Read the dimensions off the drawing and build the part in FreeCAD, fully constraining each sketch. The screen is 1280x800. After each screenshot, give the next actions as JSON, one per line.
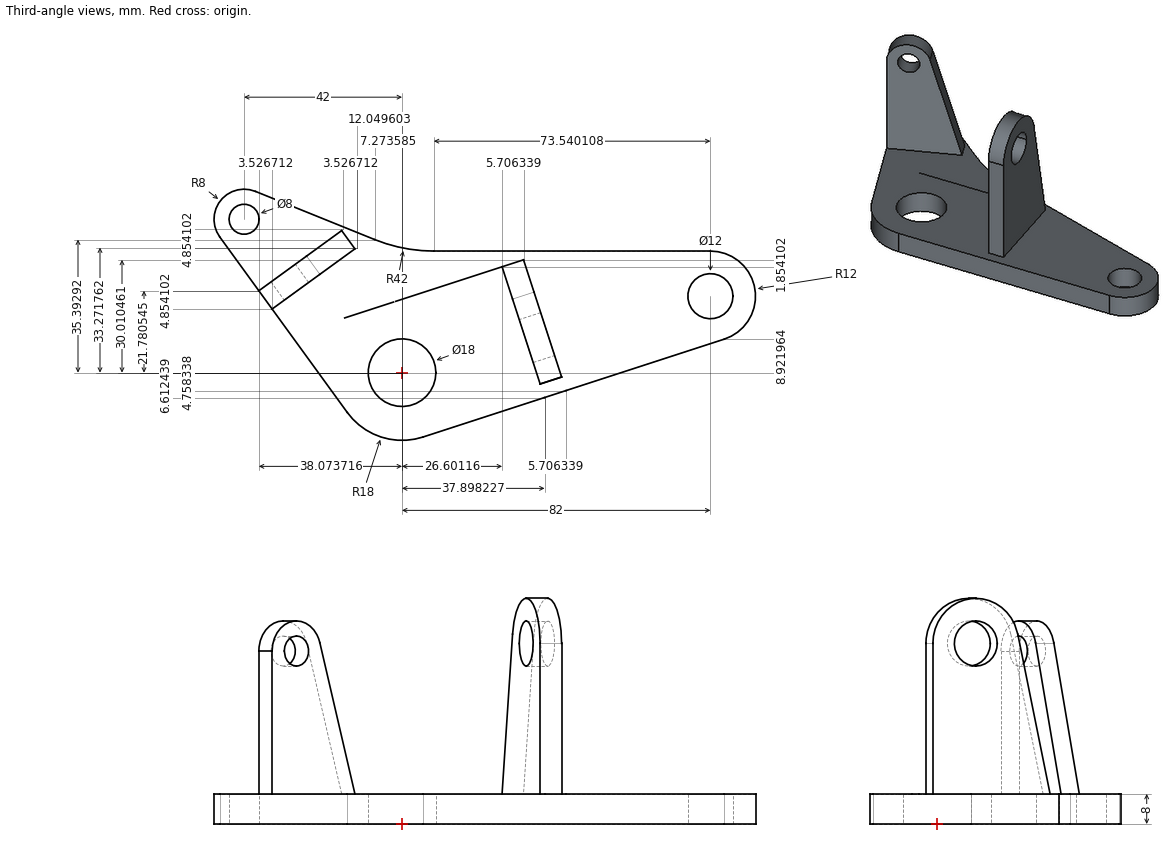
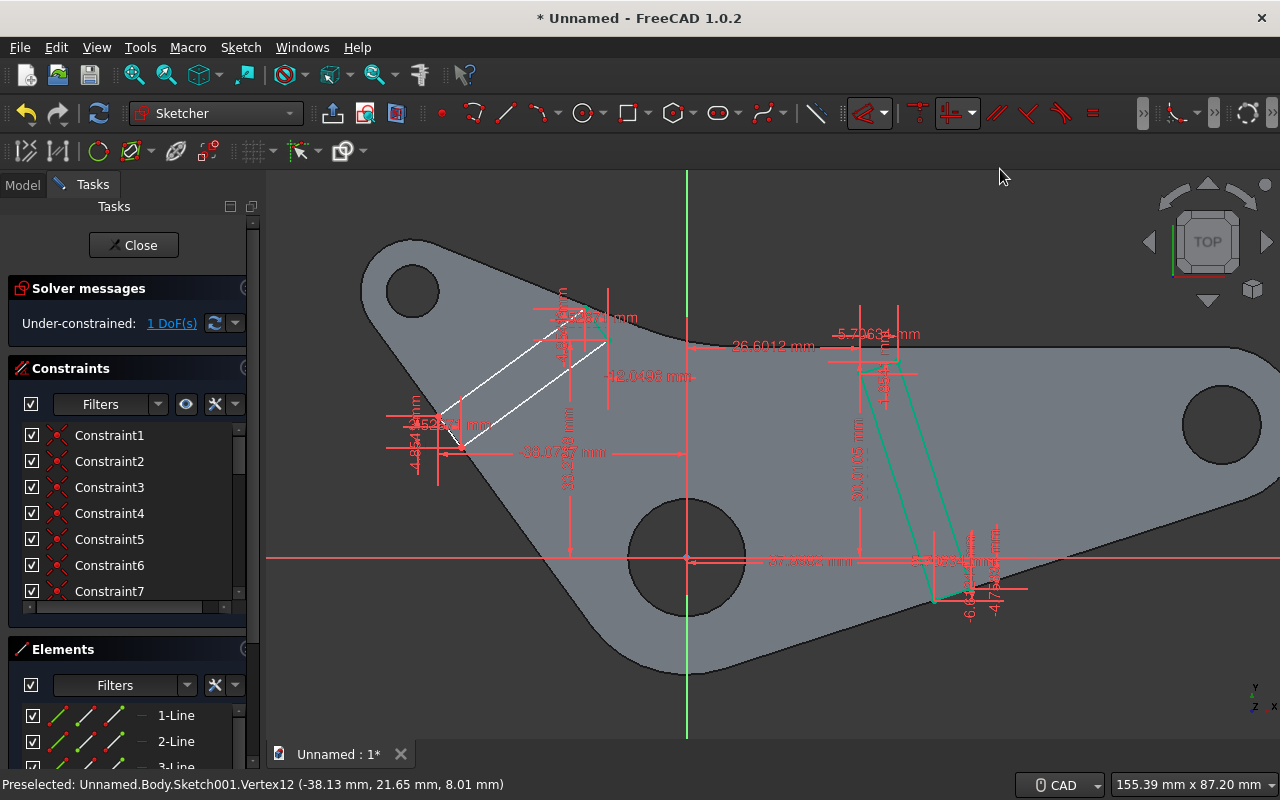
{"action": "left_click", "coordinate": [438, 416]}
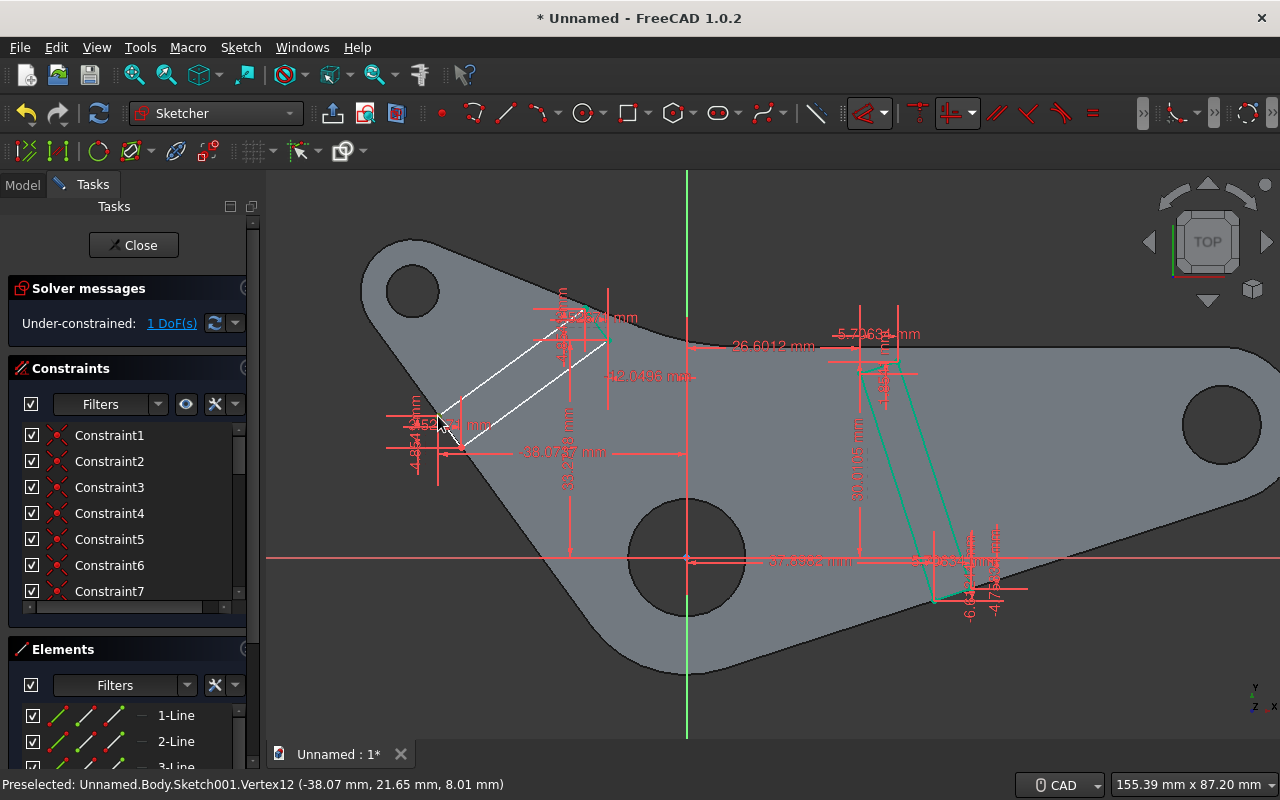
{"action": "key", "text": "i"}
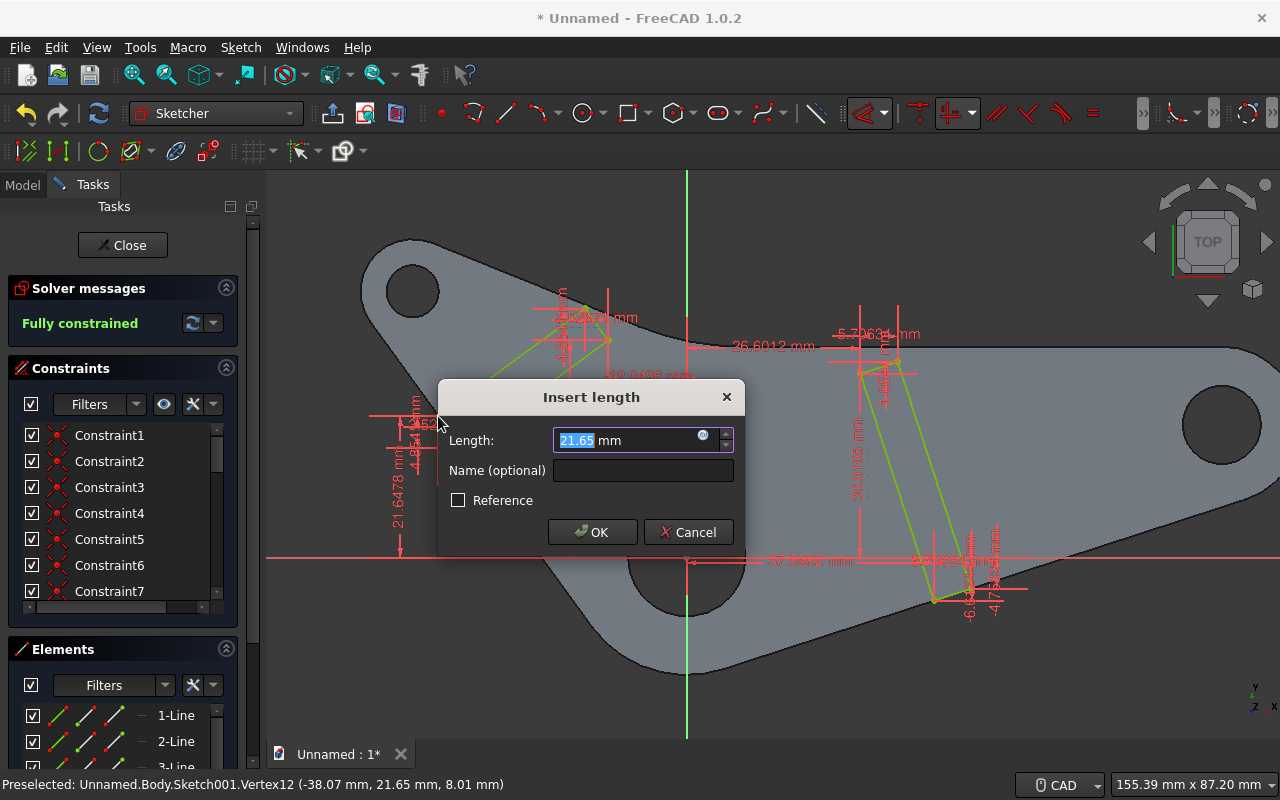
{"action": "type", "text": "21.780545"}
{"action": "key", "text": "Return"}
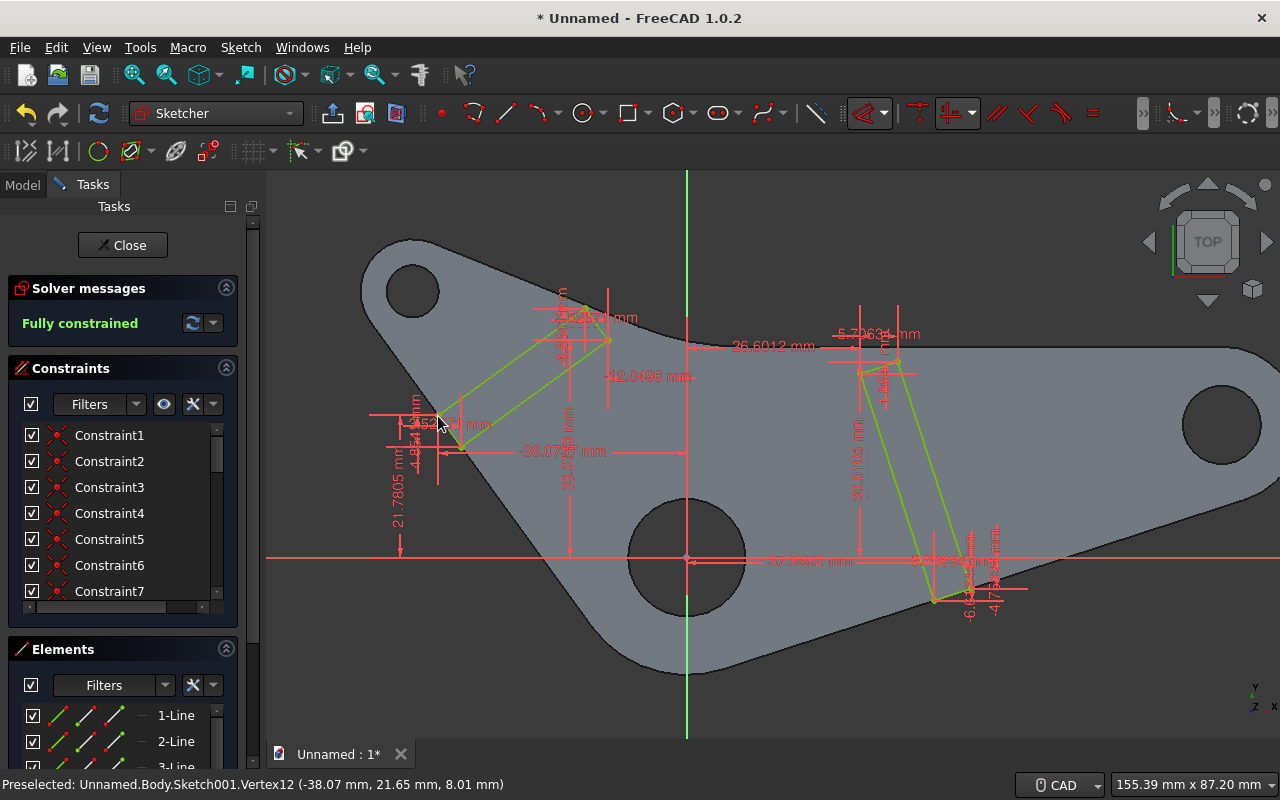
{"action": "left_click", "coordinate": [123, 245]}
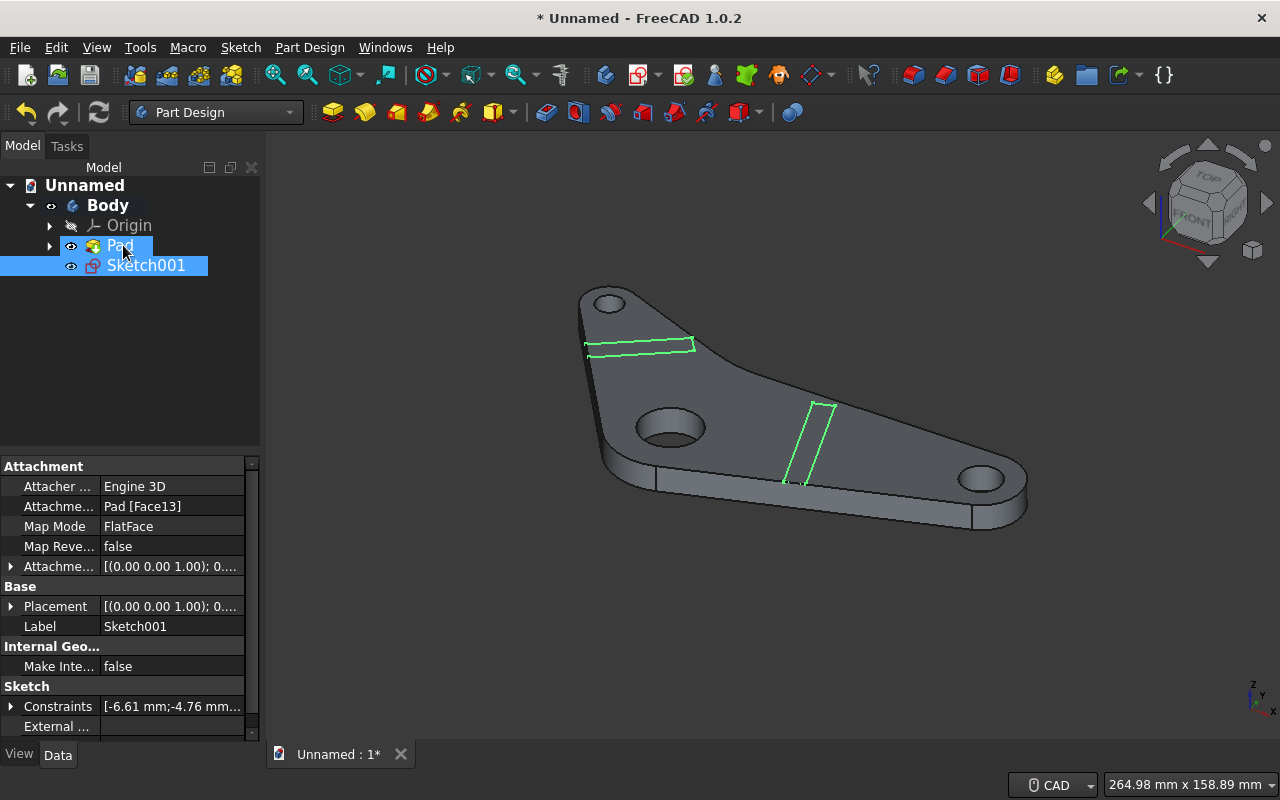
{"action": "left_click", "coordinate": [334, 112]}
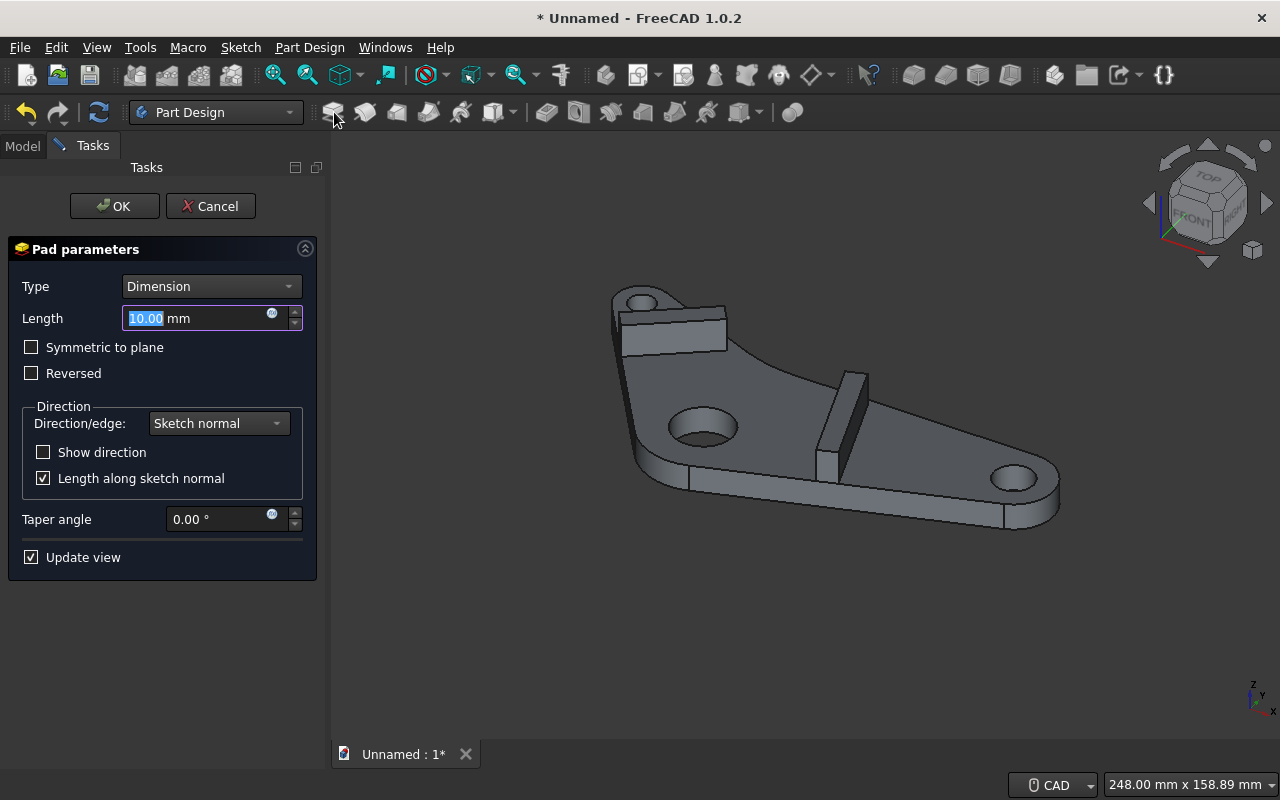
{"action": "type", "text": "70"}
{"action": "key", "text": "Tab"}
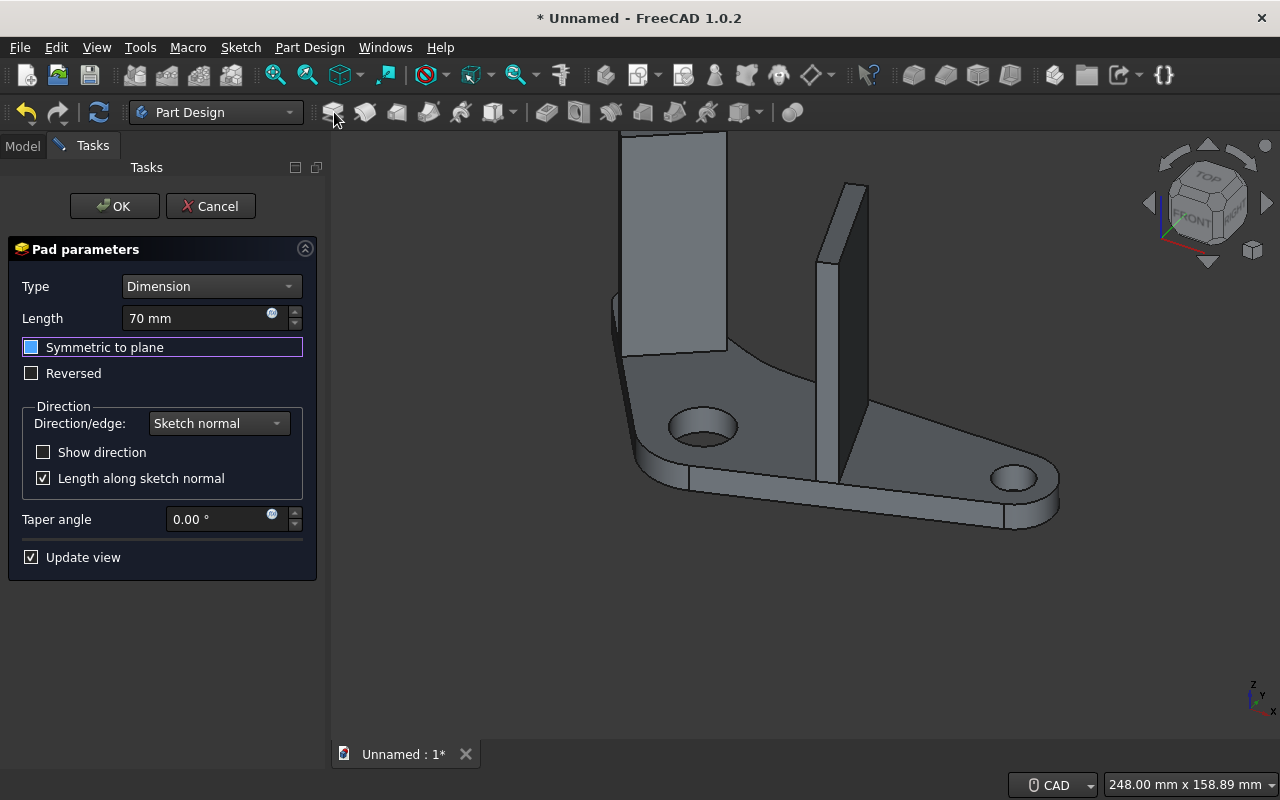
{"action": "left_click", "coordinate": [115, 206]}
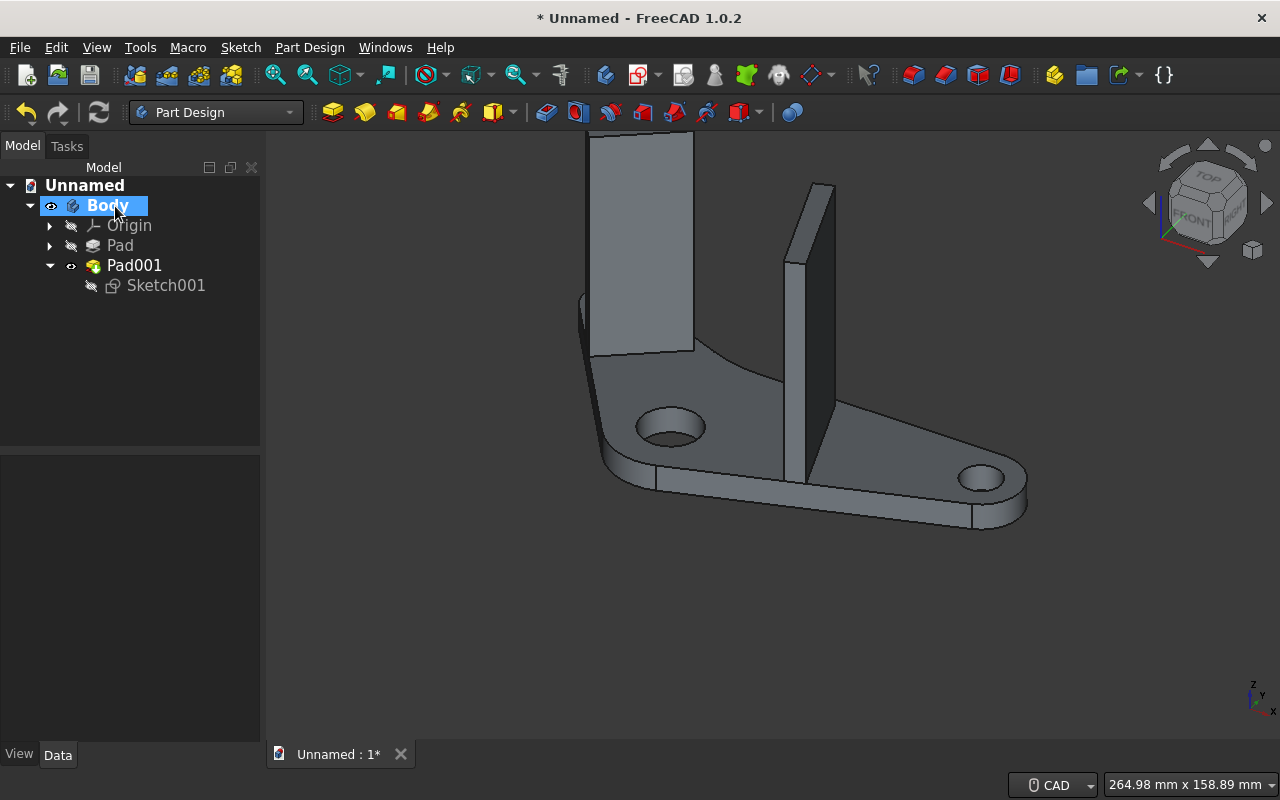
{"action": "key", "text": "v f"}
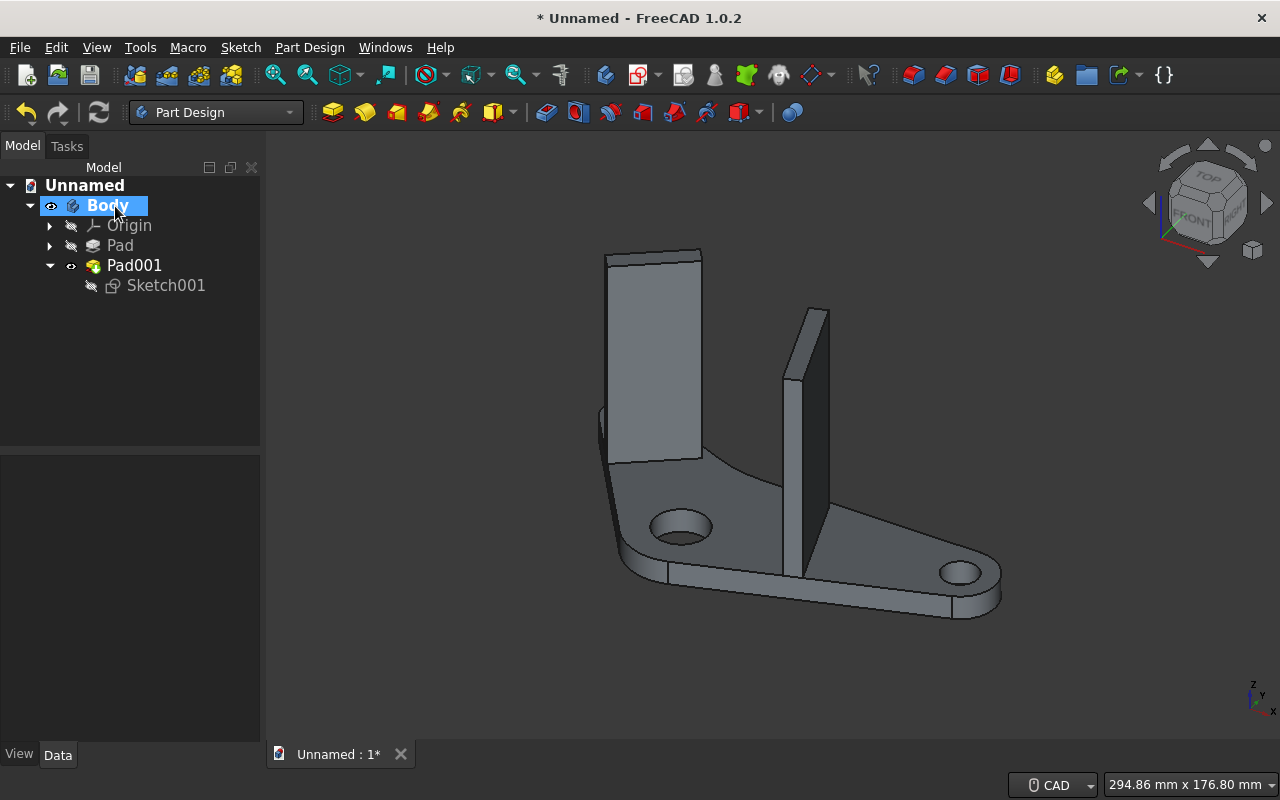
{"action": "left_click", "coordinate": [816, 415]}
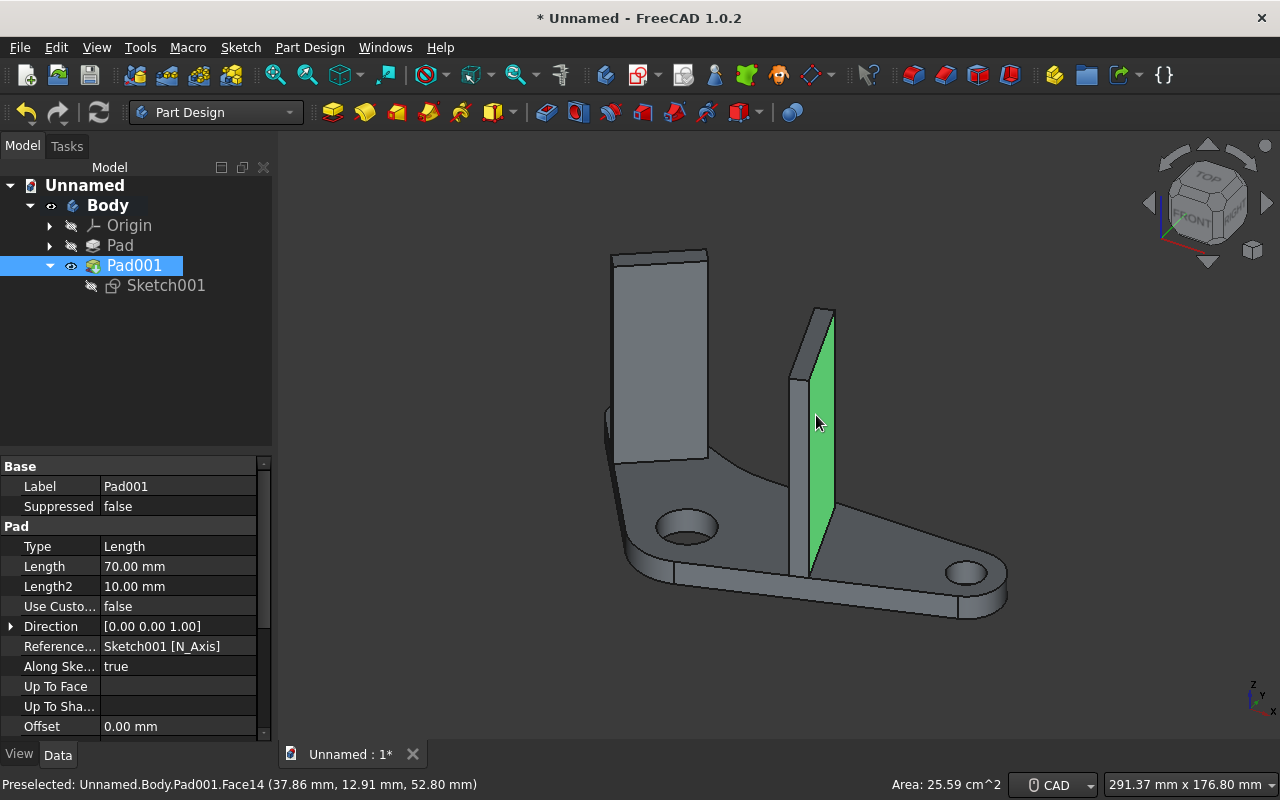
{"action": "left_click", "coordinate": [638, 76]}